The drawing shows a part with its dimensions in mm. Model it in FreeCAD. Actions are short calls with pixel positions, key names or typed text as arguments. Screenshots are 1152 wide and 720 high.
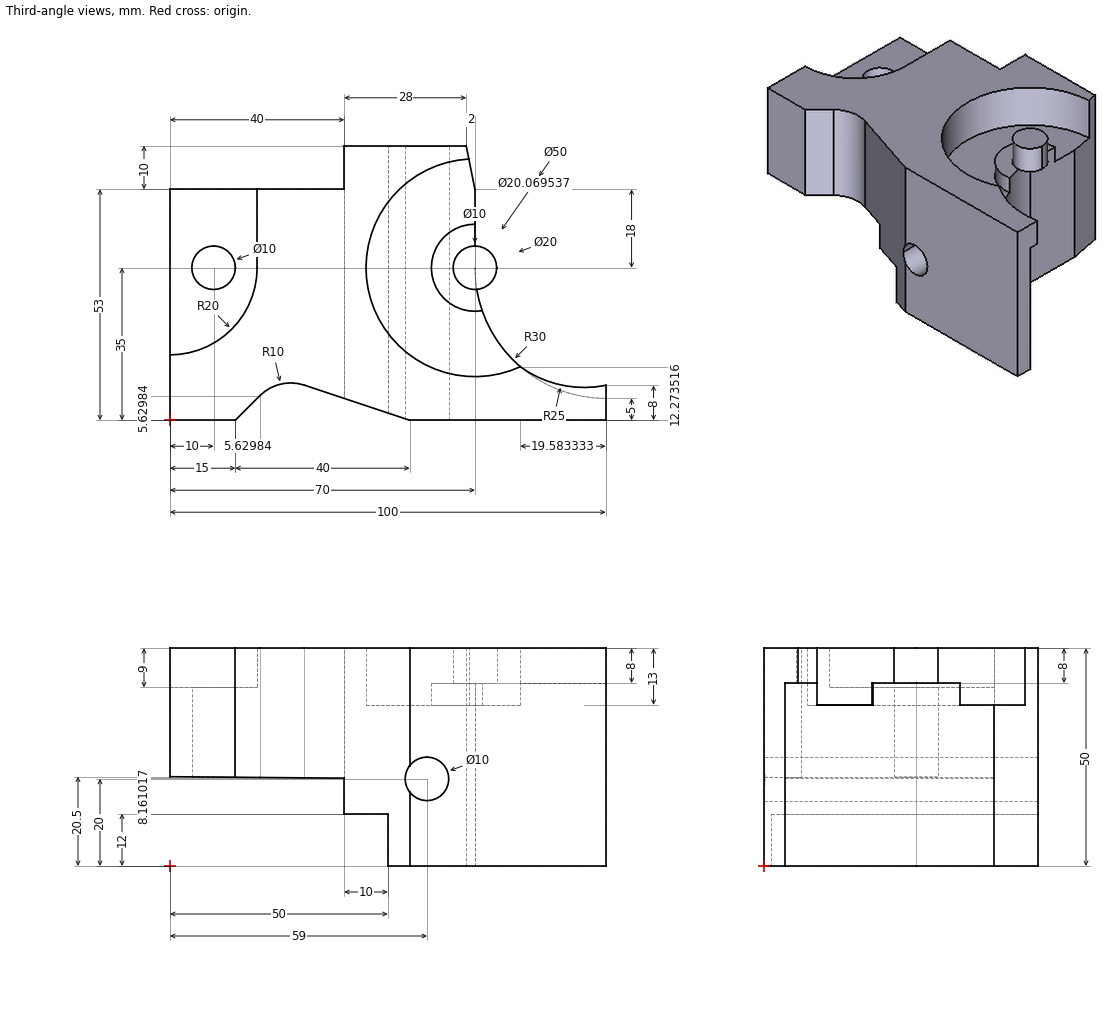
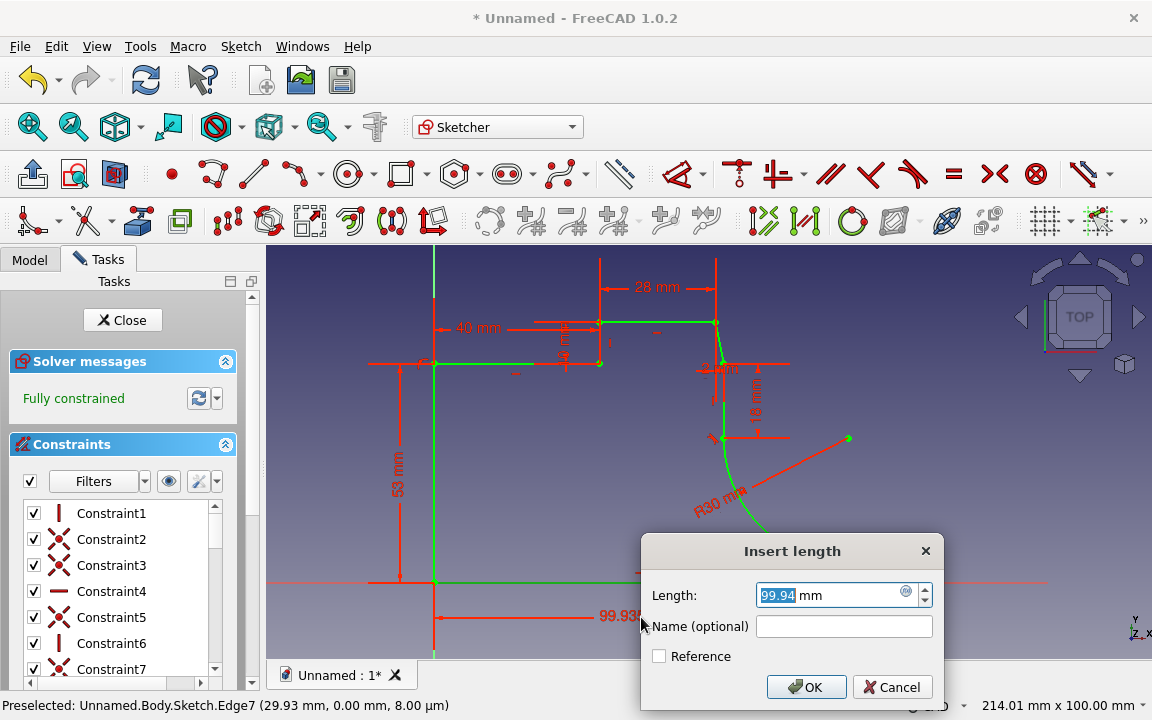
text(100)
key(Return)
key(Escape)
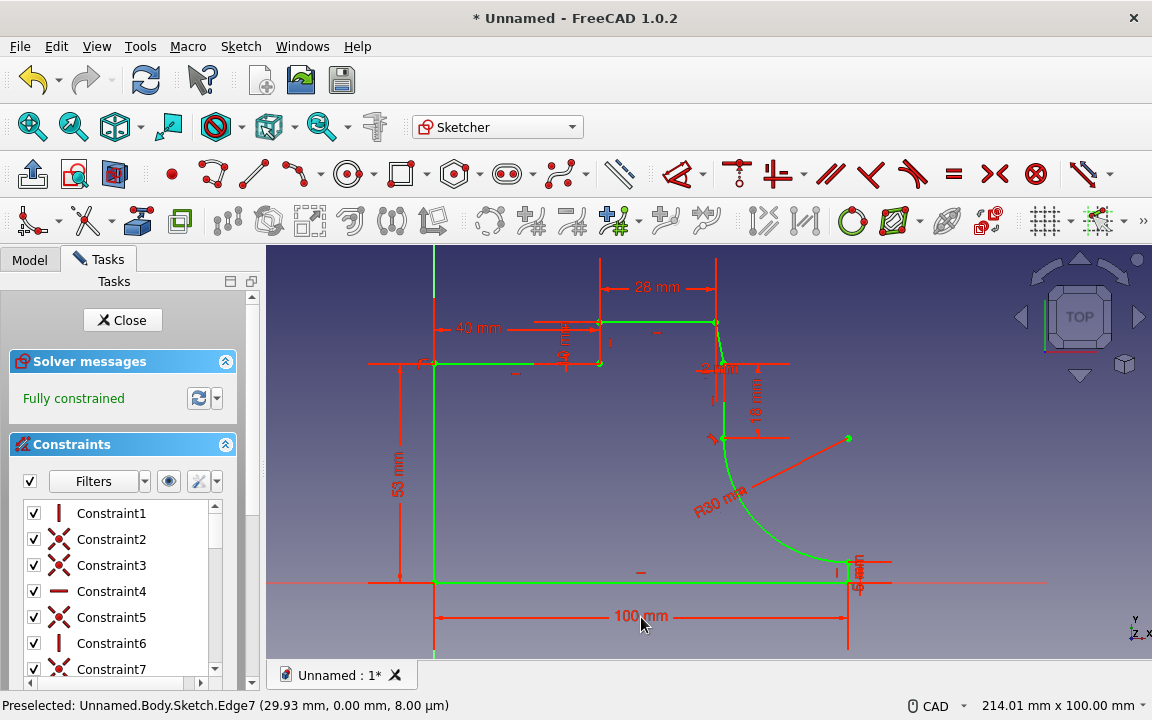
click(123, 320)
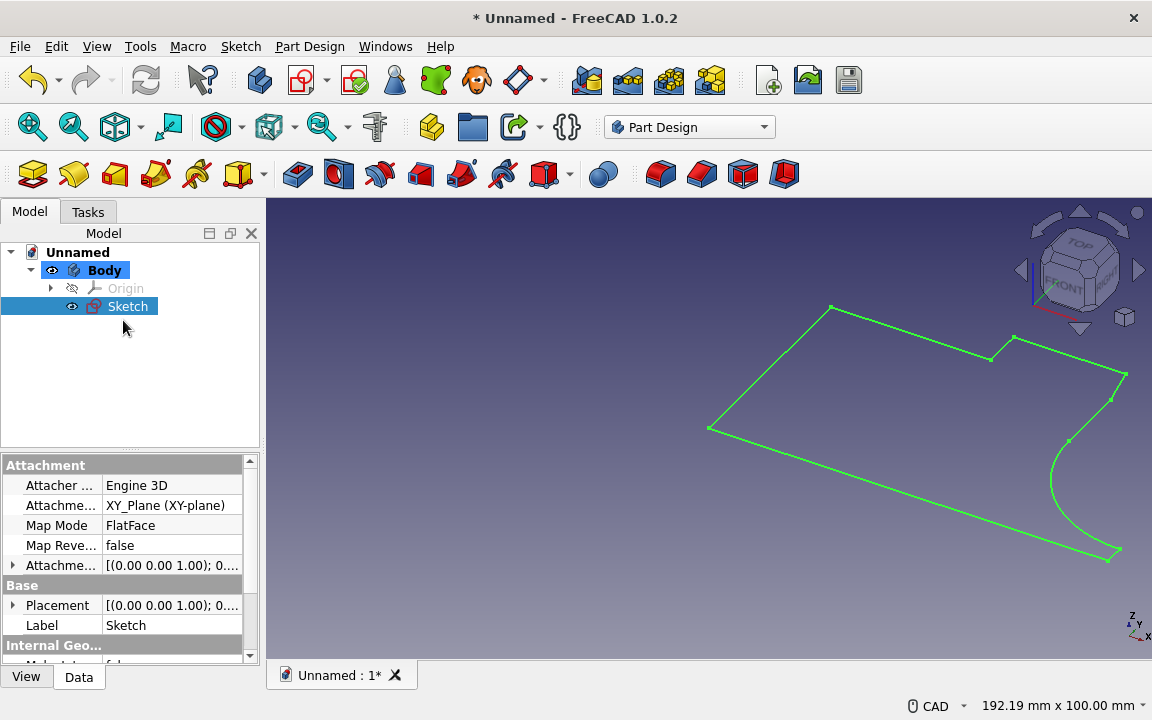
click(33, 174)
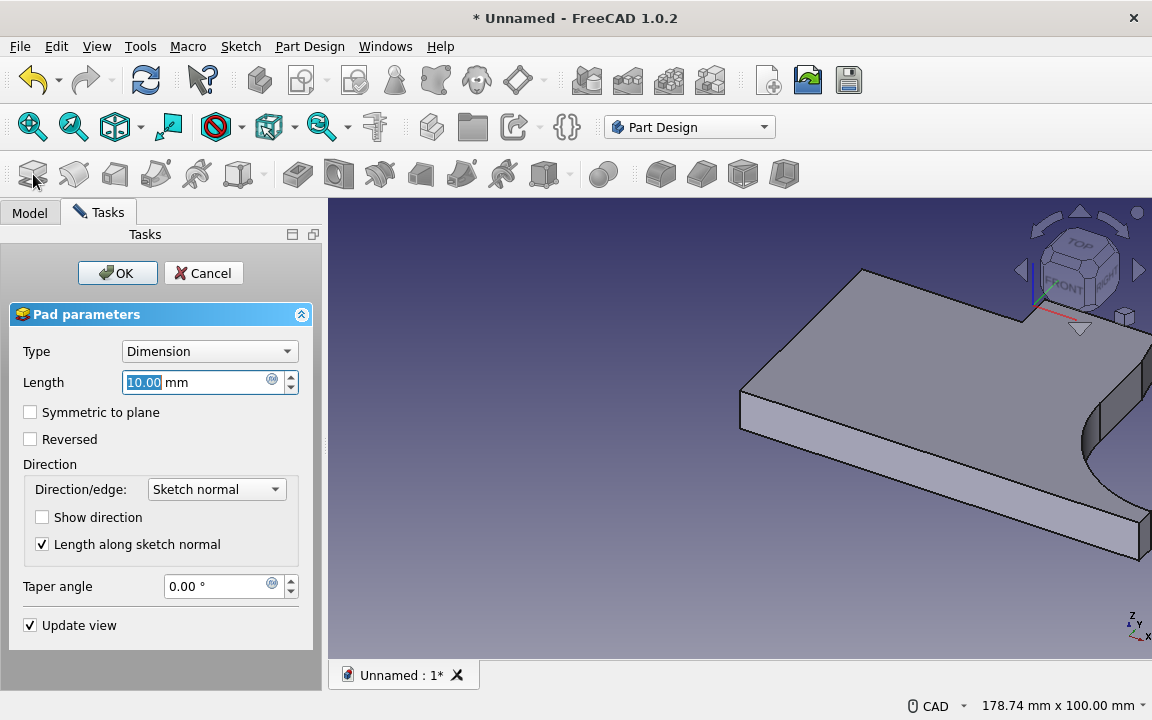
text(50)
key(Tab)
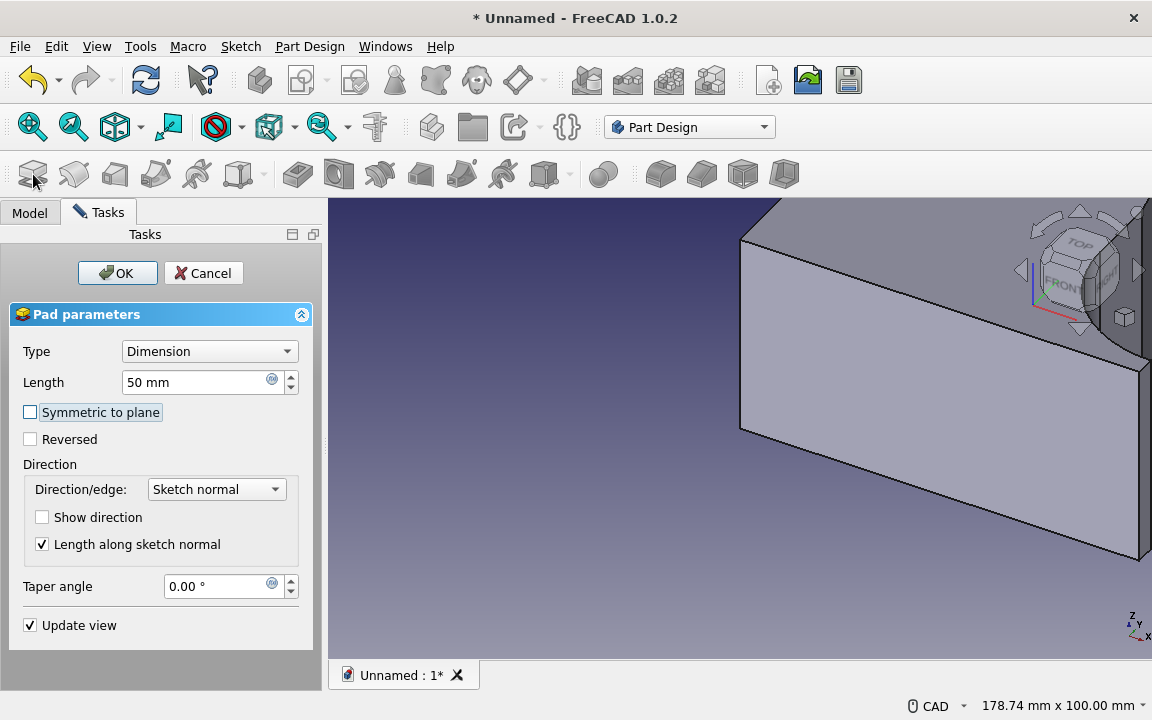
click(118, 273)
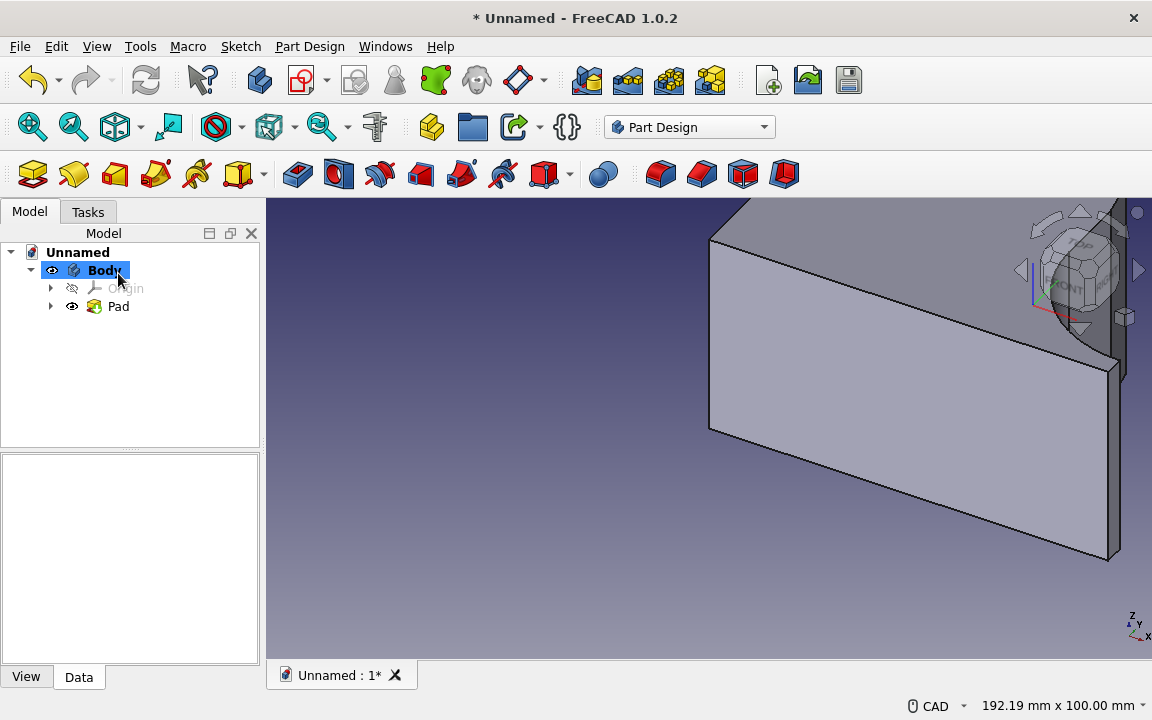
key(v)
key(f)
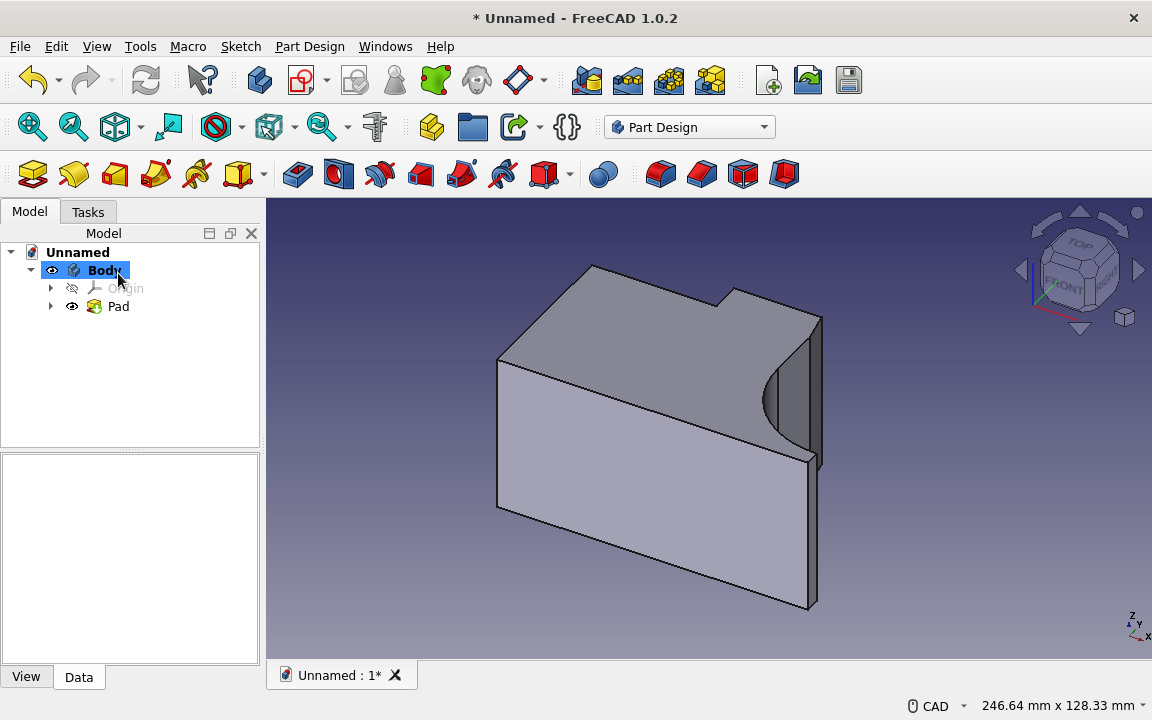
click(51, 288)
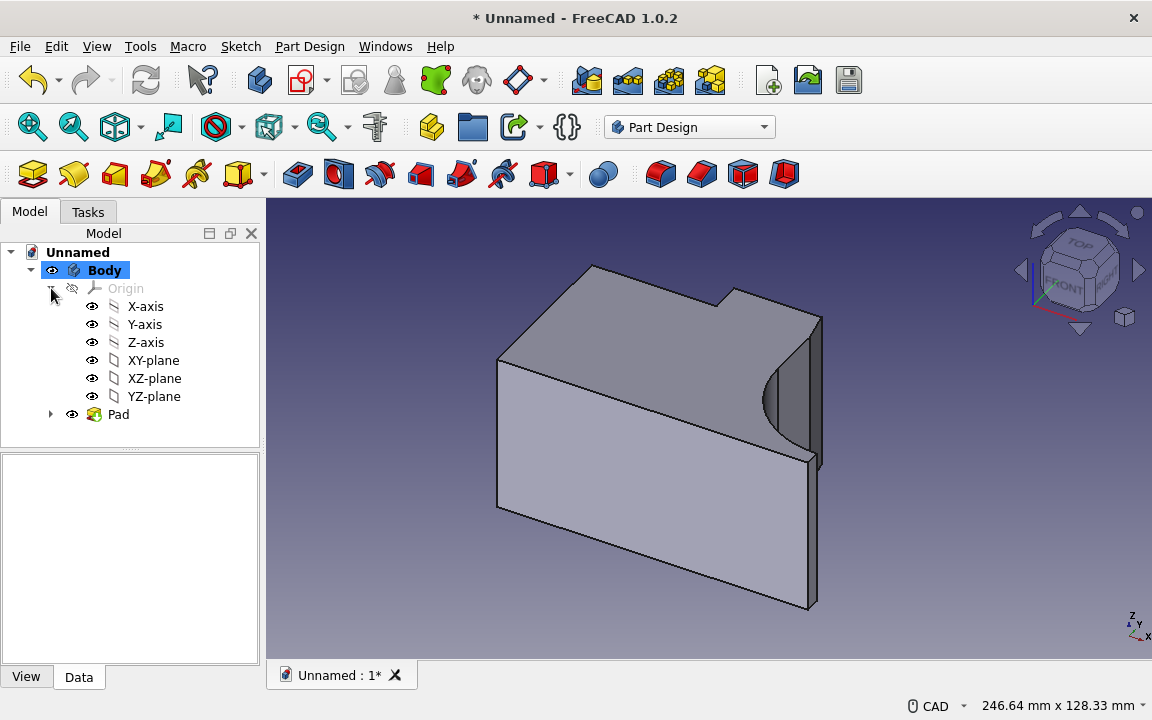
click(137, 360)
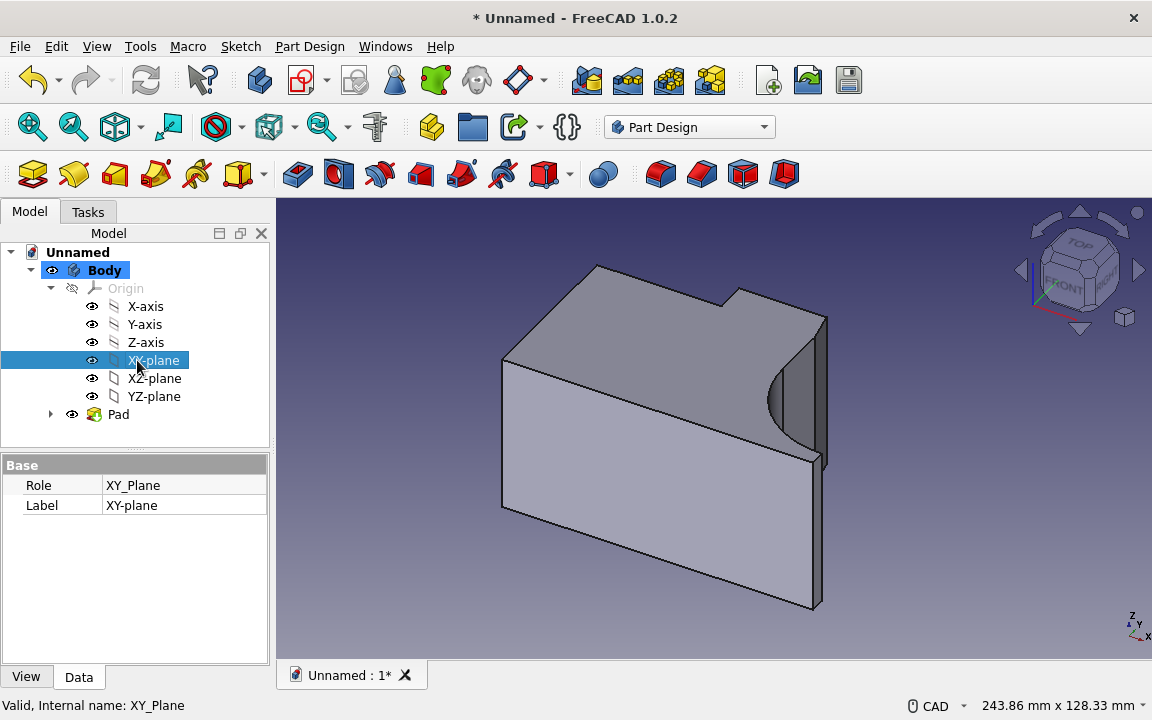
click(518, 80)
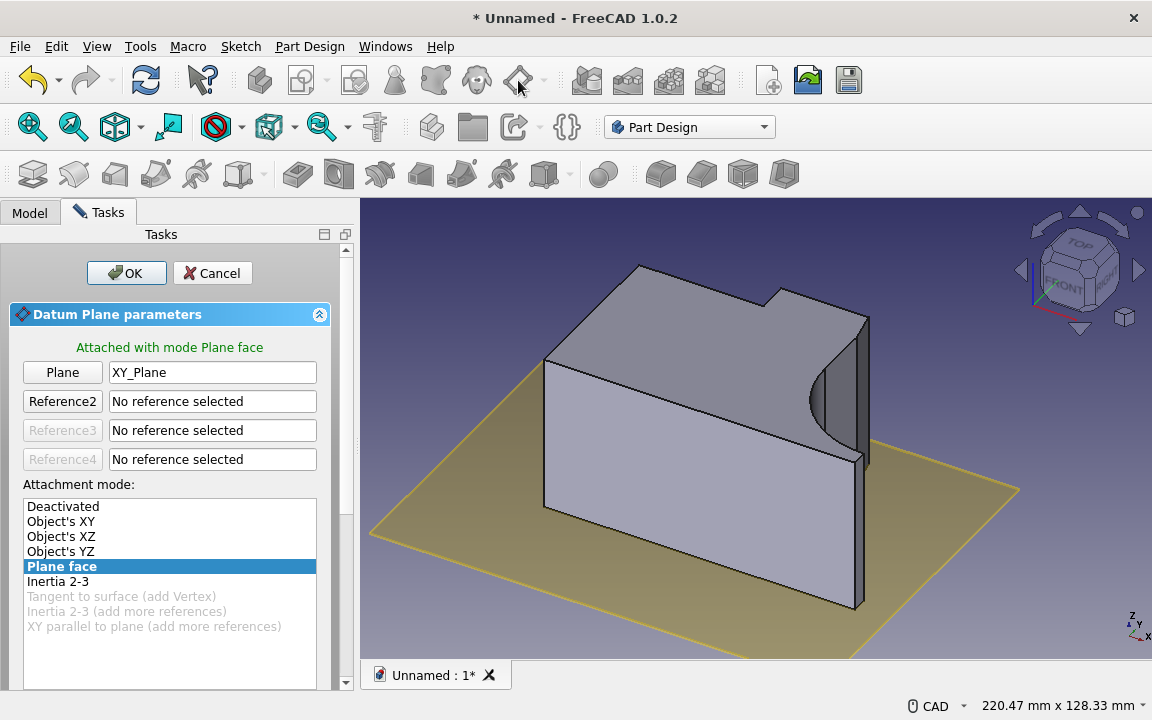
scroll(346, 467, down, 4)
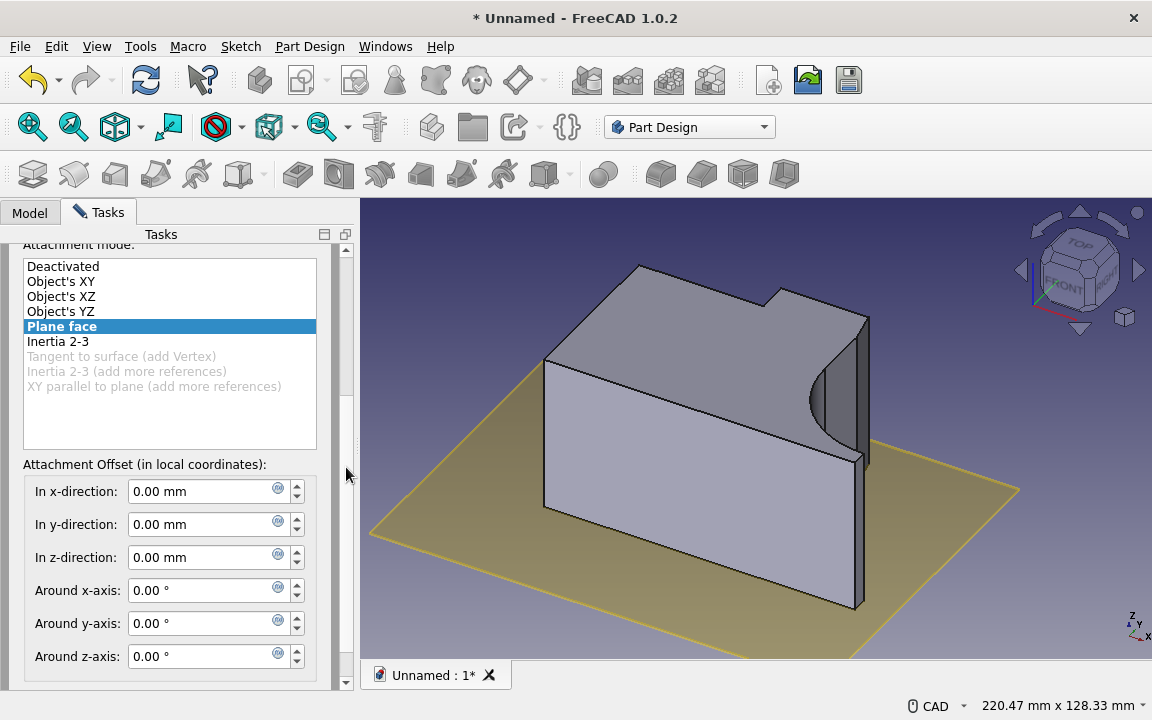
triple_click(210, 558)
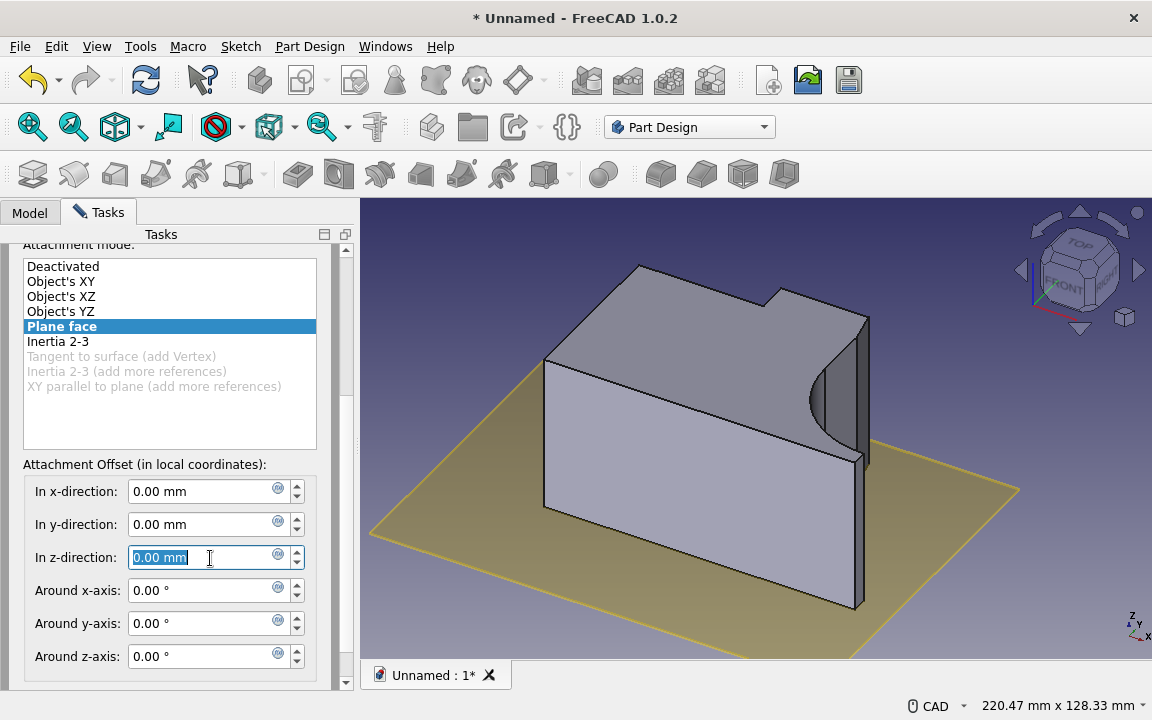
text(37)
key(Tab)